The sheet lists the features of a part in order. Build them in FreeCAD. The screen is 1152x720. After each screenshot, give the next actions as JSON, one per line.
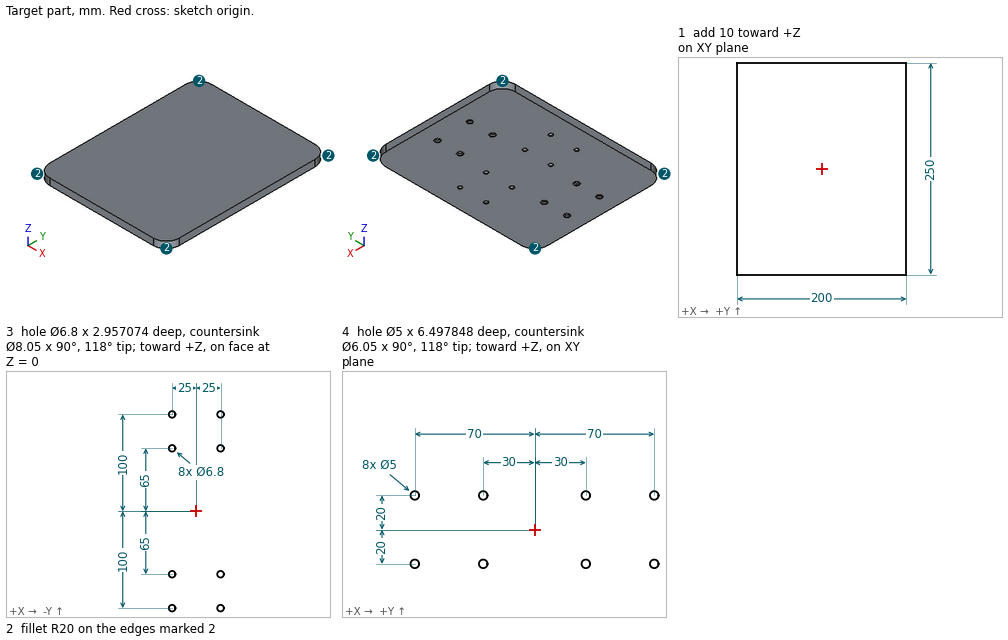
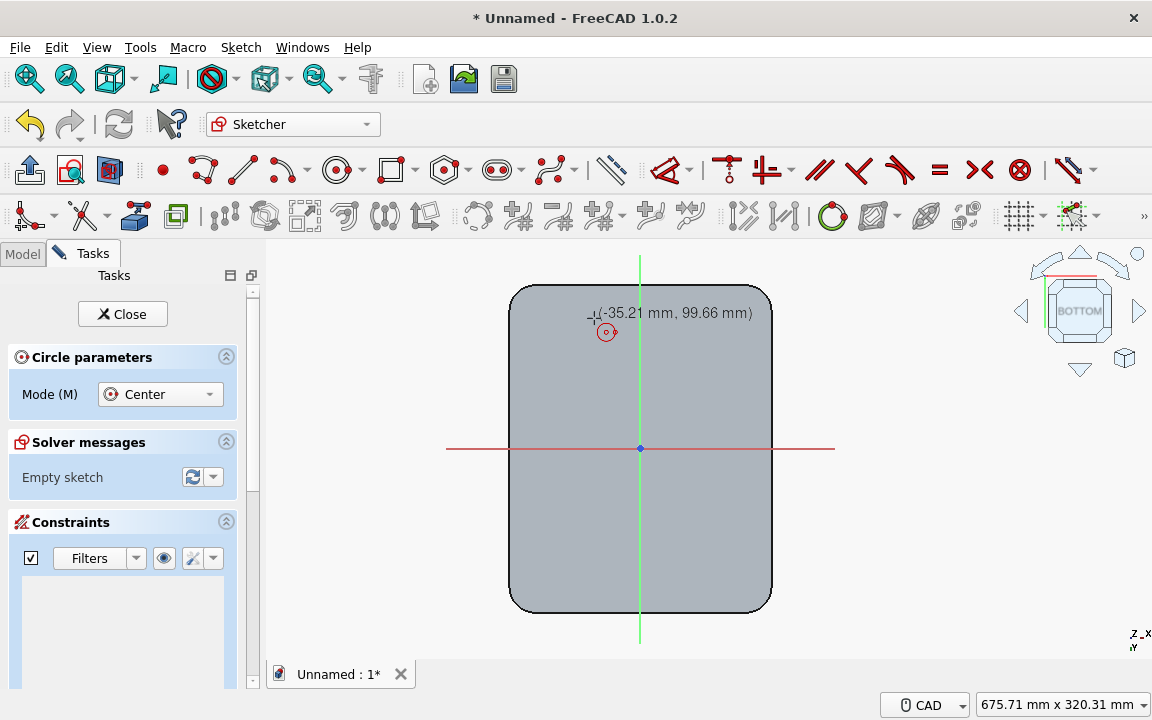
{"action": "left_click", "coordinate": [608, 318]}
{"action": "mouse_move", "coordinate": [611, 315]}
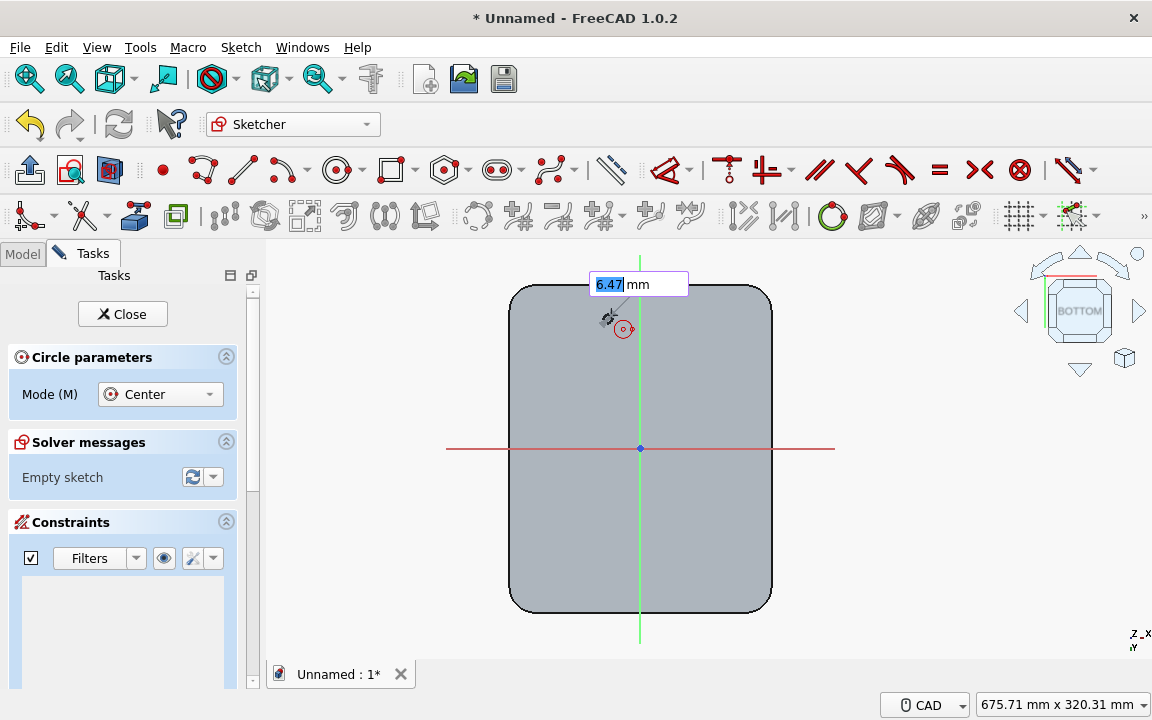
{"action": "type", "text": "6.8"}
{"action": "key", "text": "Return"}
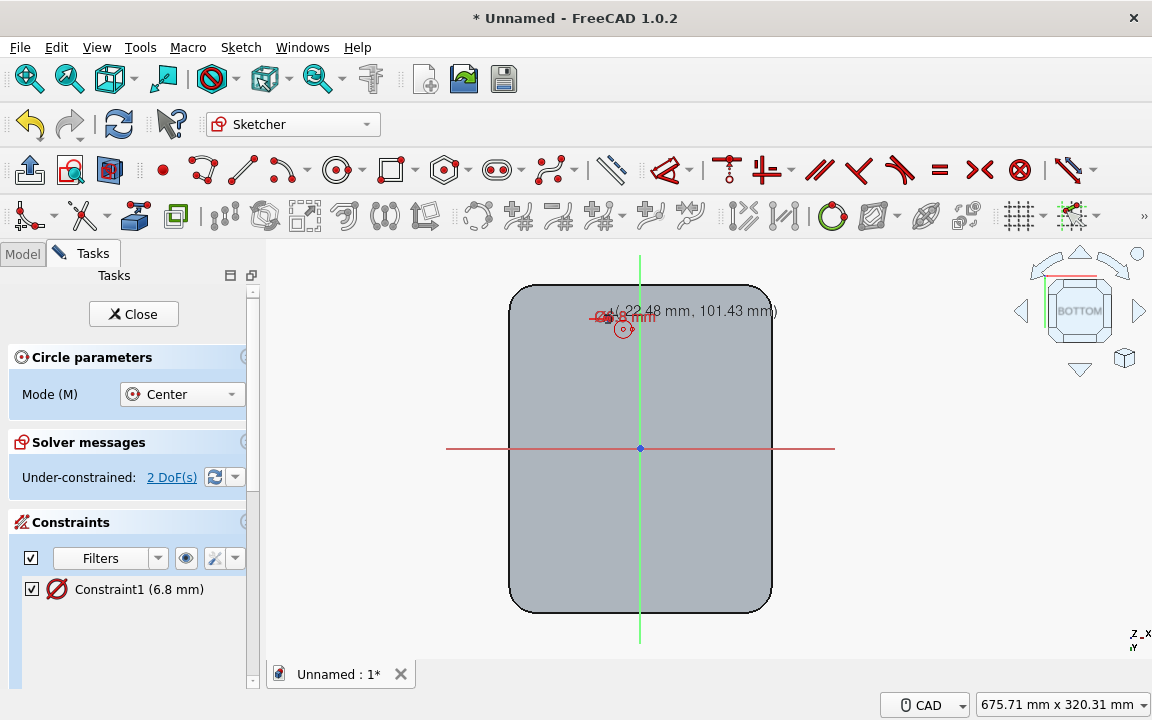
{"action": "scroll", "coordinate": [608, 364], "scroll_direction": "up", "scroll_amount": 9}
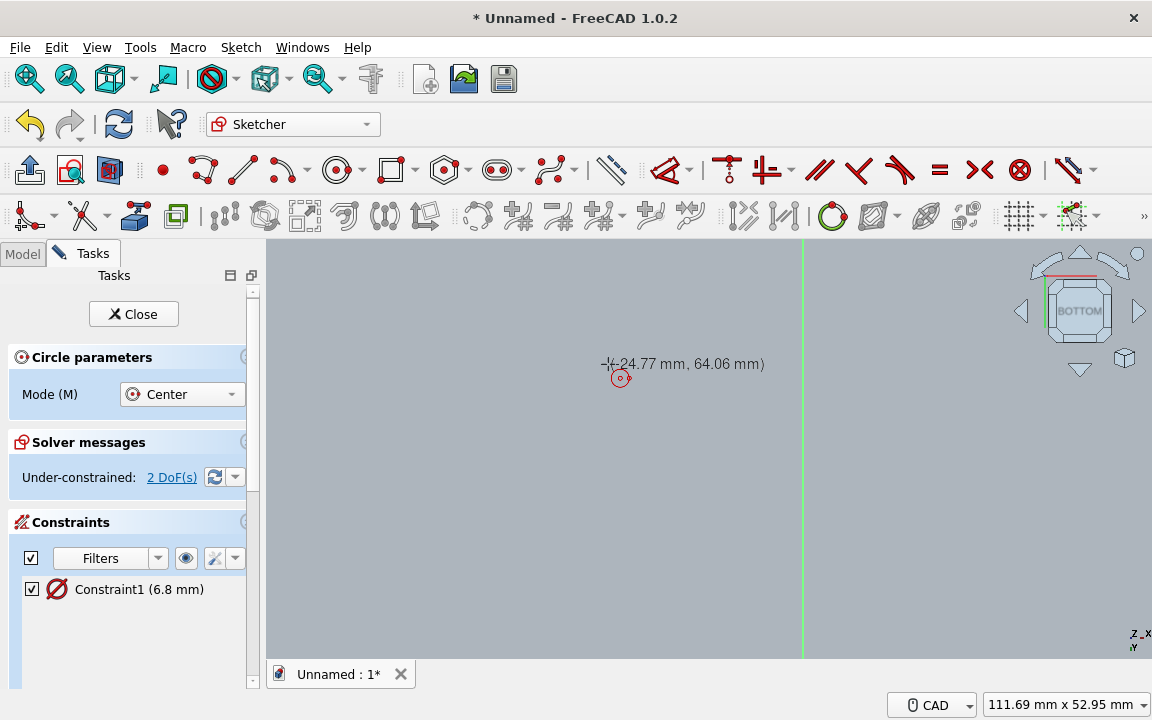
{"action": "scroll", "coordinate": [608, 364], "scroll_direction": "down", "scroll_amount": 9}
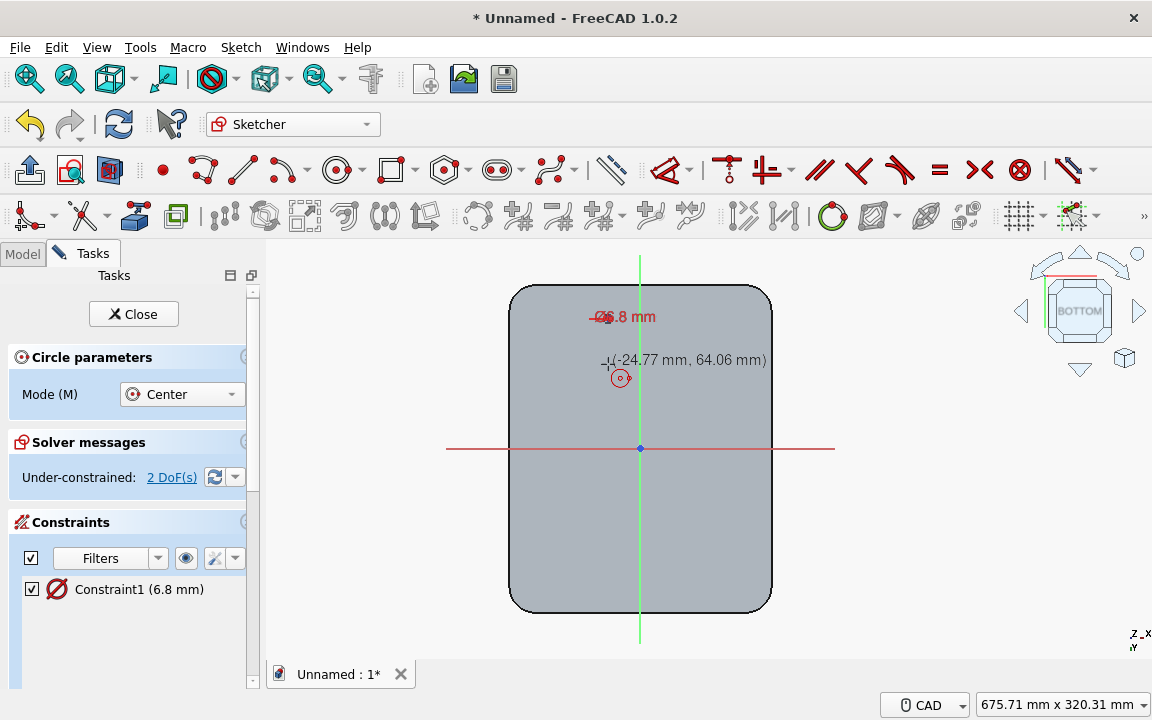
{"action": "left_click", "coordinate": [608, 364]}
{"action": "mouse_move", "coordinate": [611, 361]}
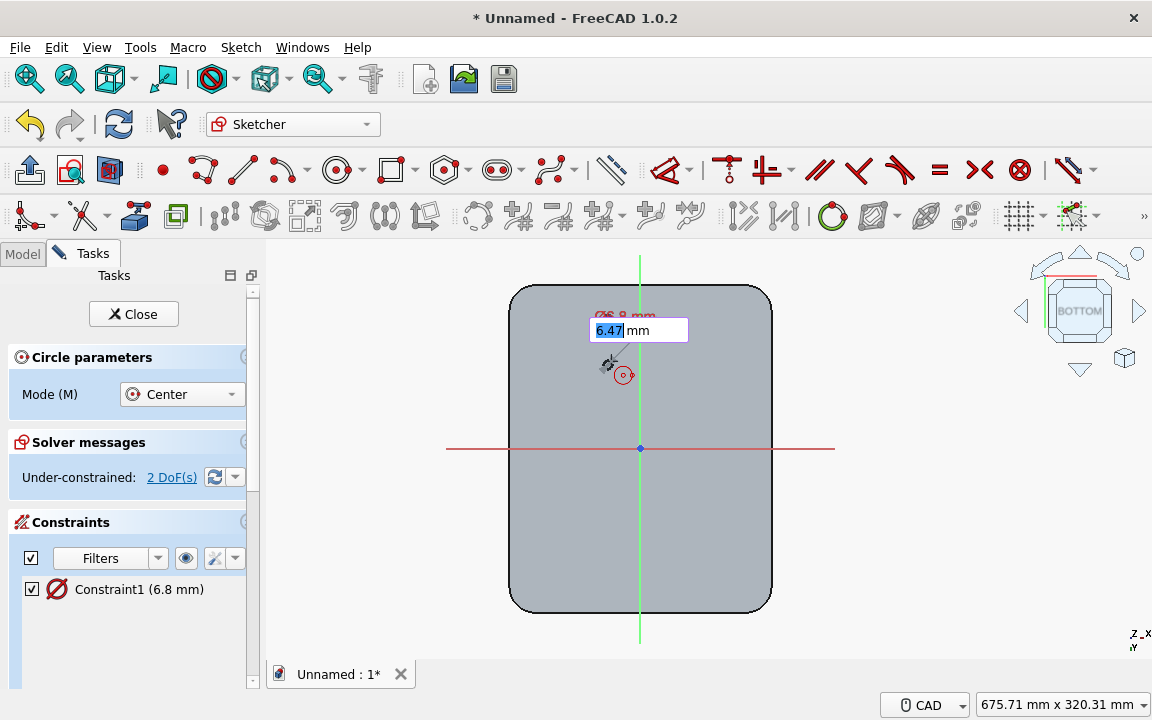
{"action": "type", "text": "6.8"}
{"action": "key", "text": "Return"}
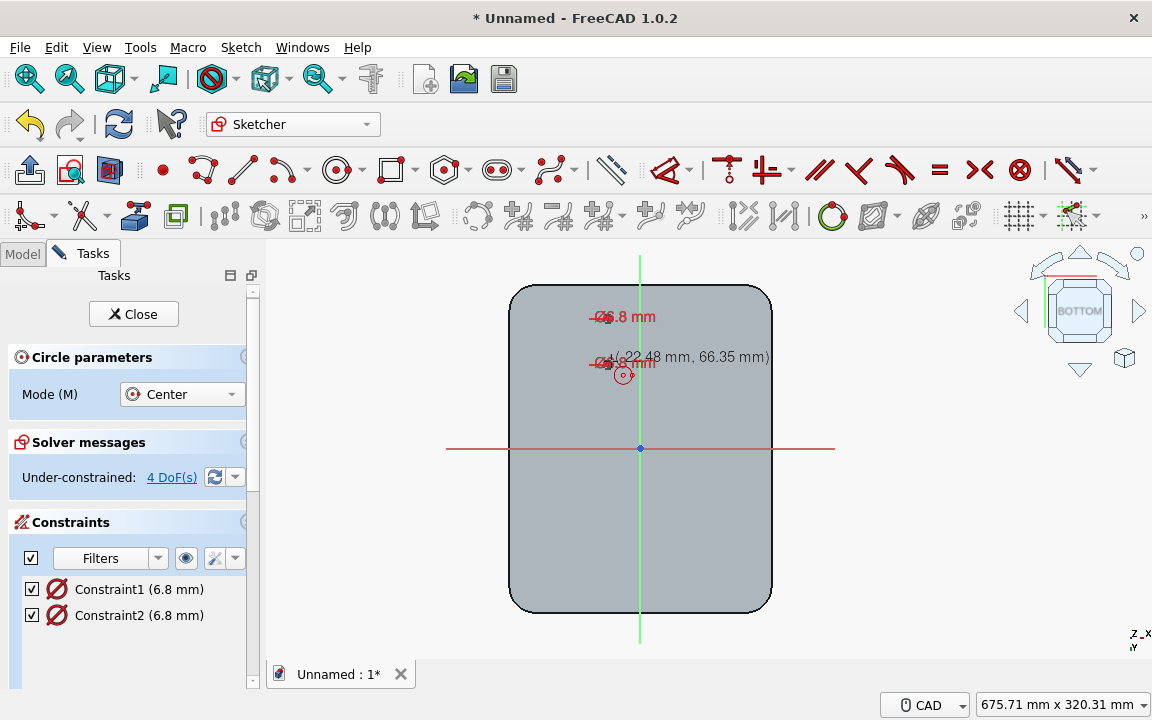
{"action": "scroll", "coordinate": [673, 364], "scroll_direction": "up", "scroll_amount": 9}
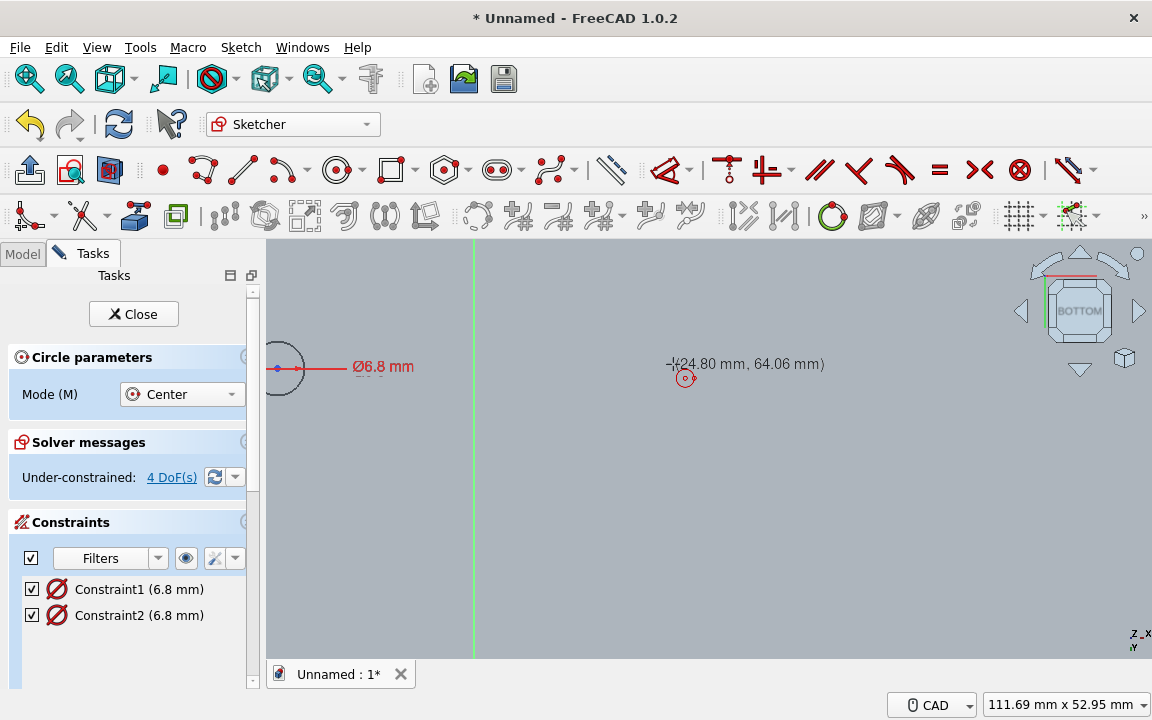
{"action": "scroll", "coordinate": [673, 364], "scroll_direction": "down", "scroll_amount": 9}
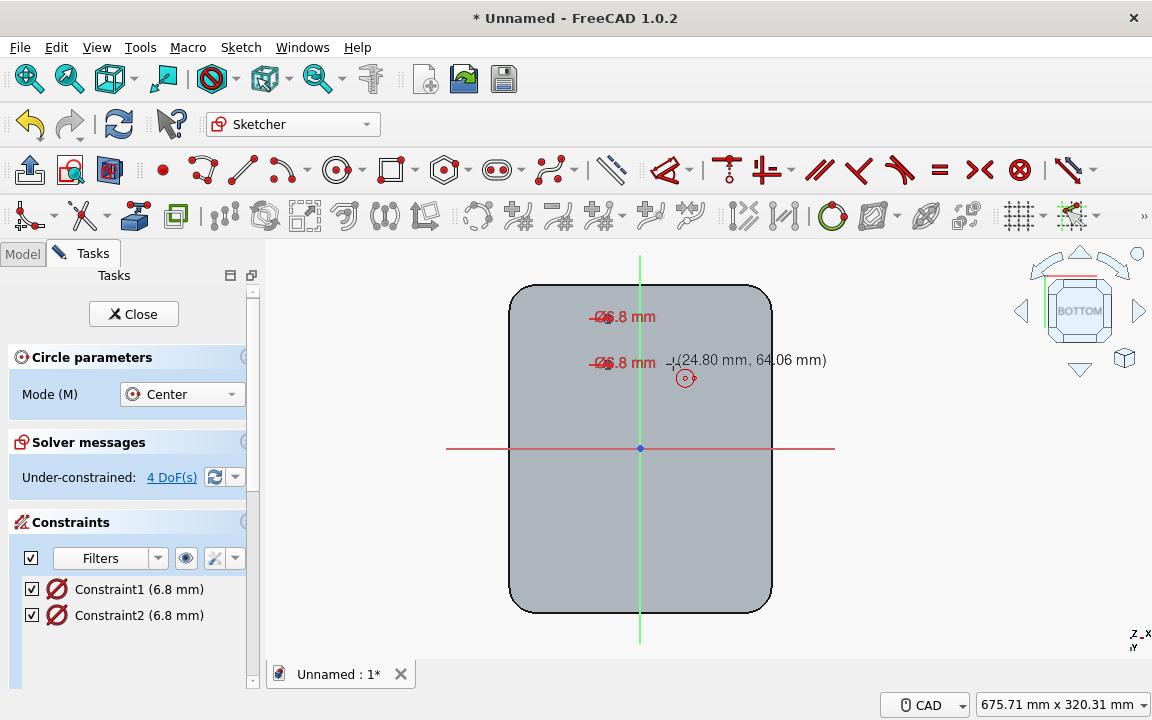
{"action": "left_click", "coordinate": [673, 364]}
{"action": "mouse_move", "coordinate": [676, 361]}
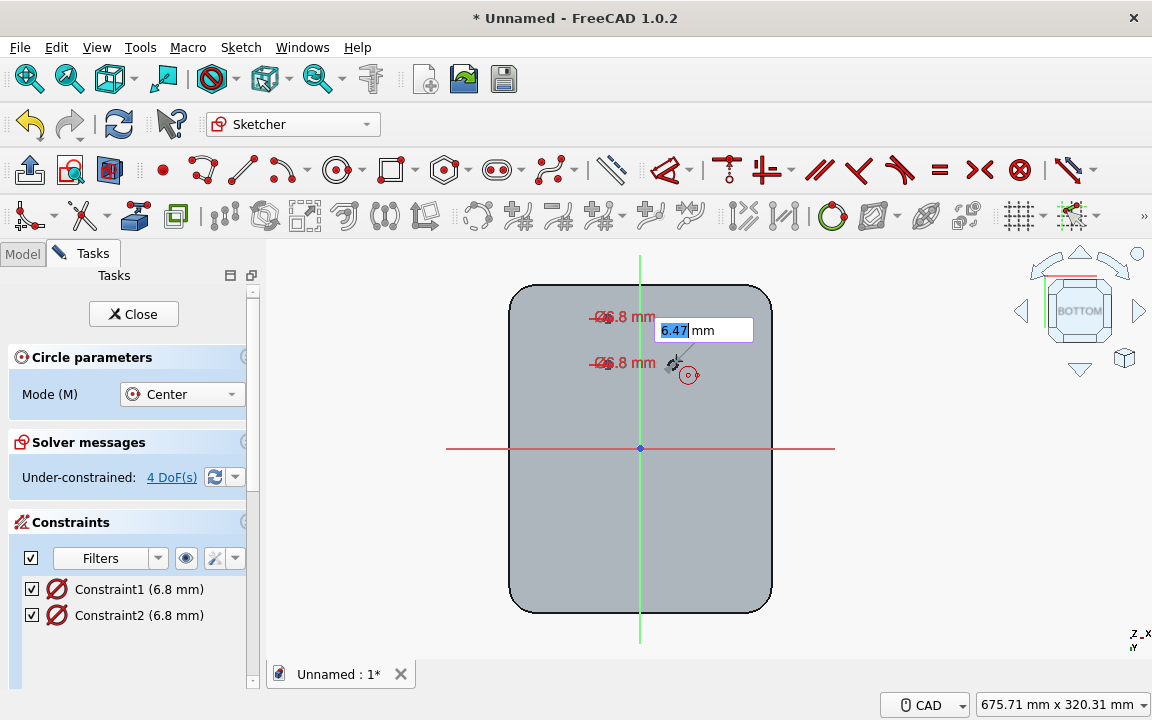
{"action": "type", "text": "6.8"}
{"action": "key", "text": "Return"}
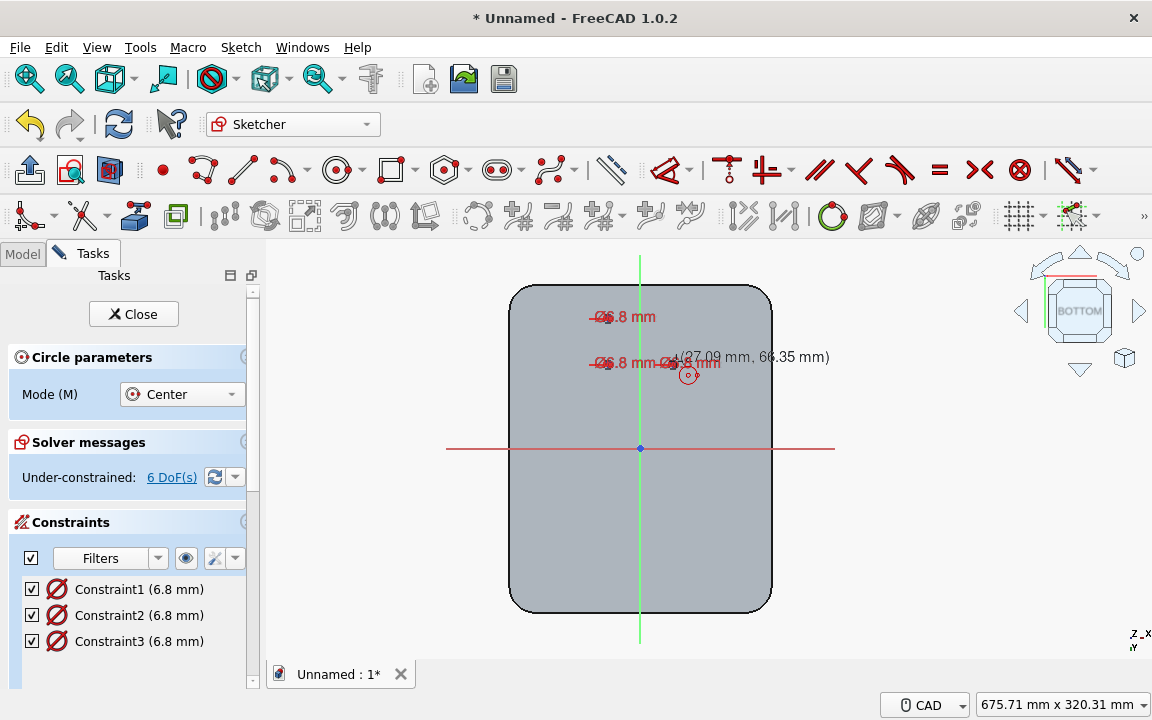
{"action": "scroll", "coordinate": [673, 318], "scroll_direction": "up", "scroll_amount": 9}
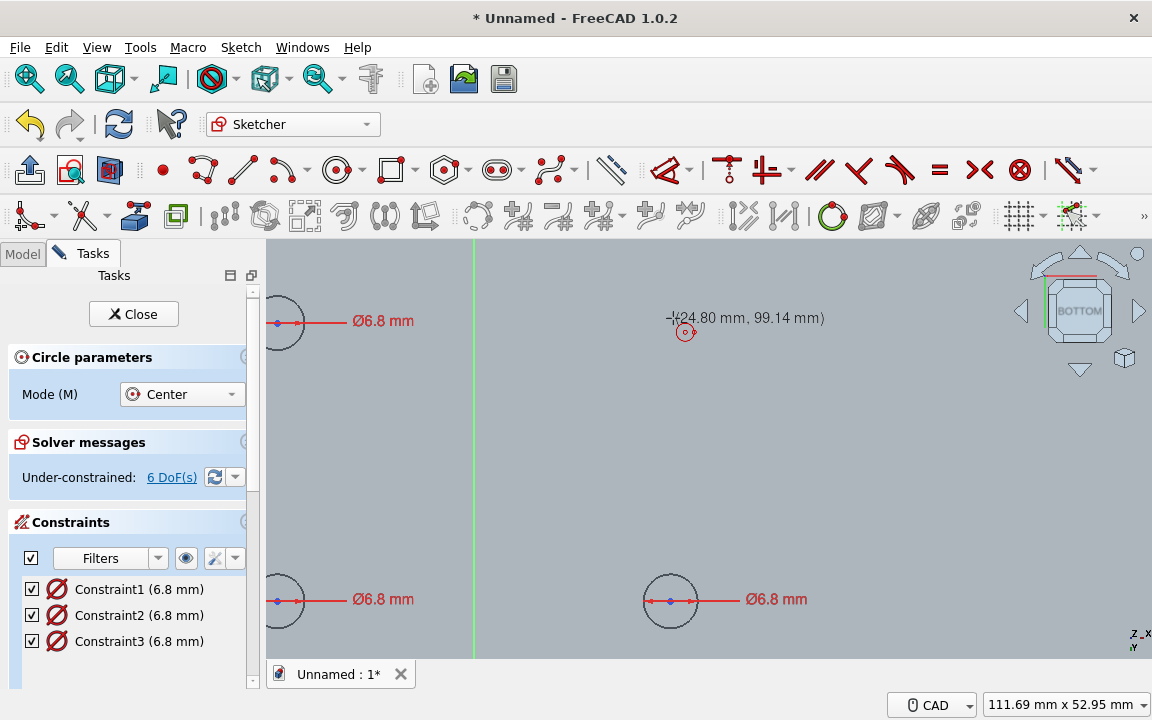
{"action": "scroll", "coordinate": [673, 318], "scroll_direction": "down", "scroll_amount": 9}